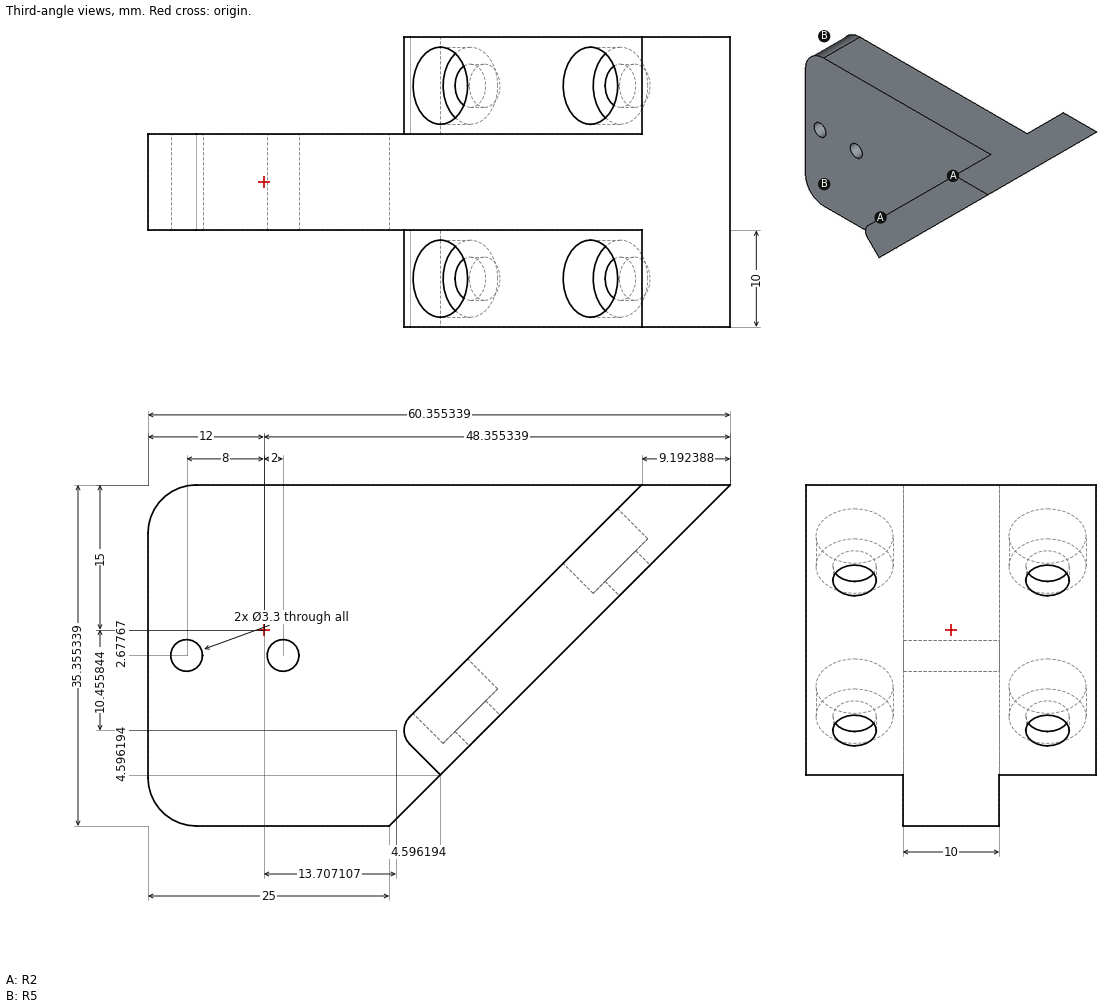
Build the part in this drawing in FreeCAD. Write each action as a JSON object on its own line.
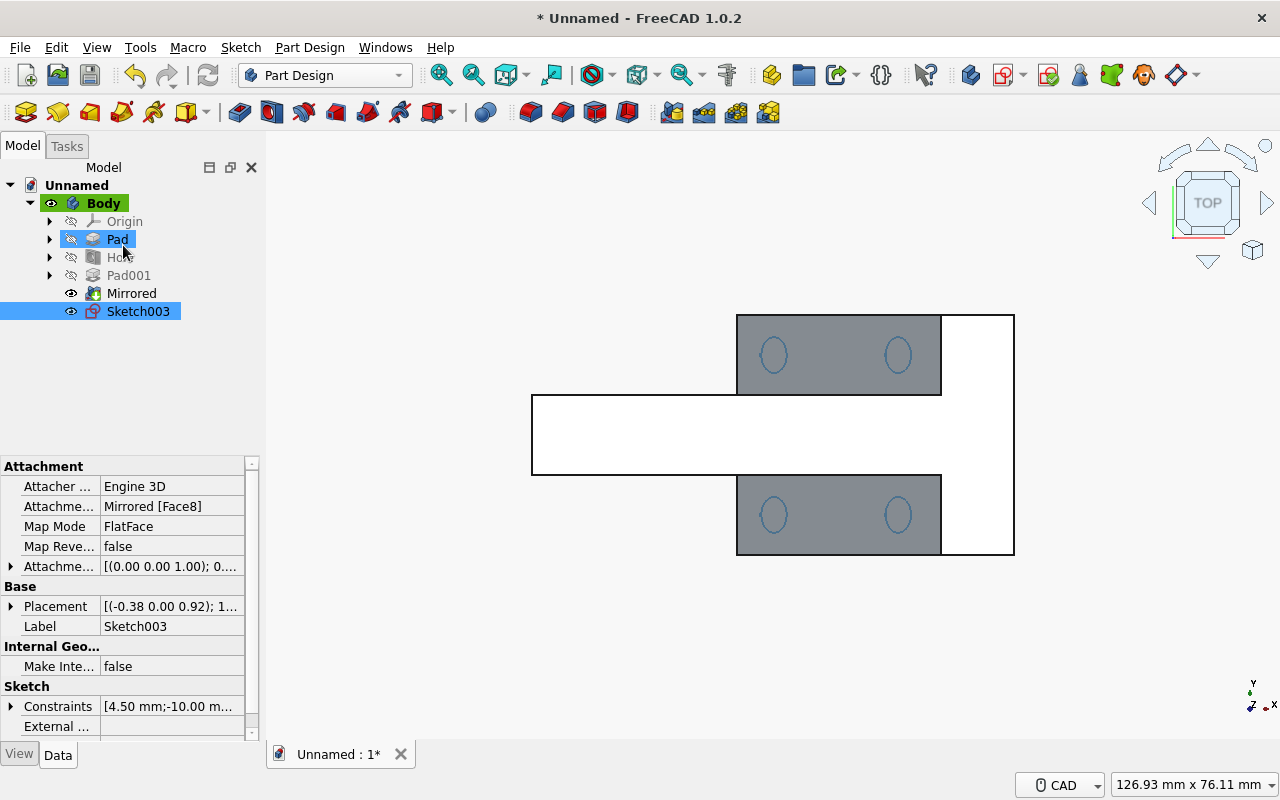
{"action": "left_click", "coordinate": [272, 112]}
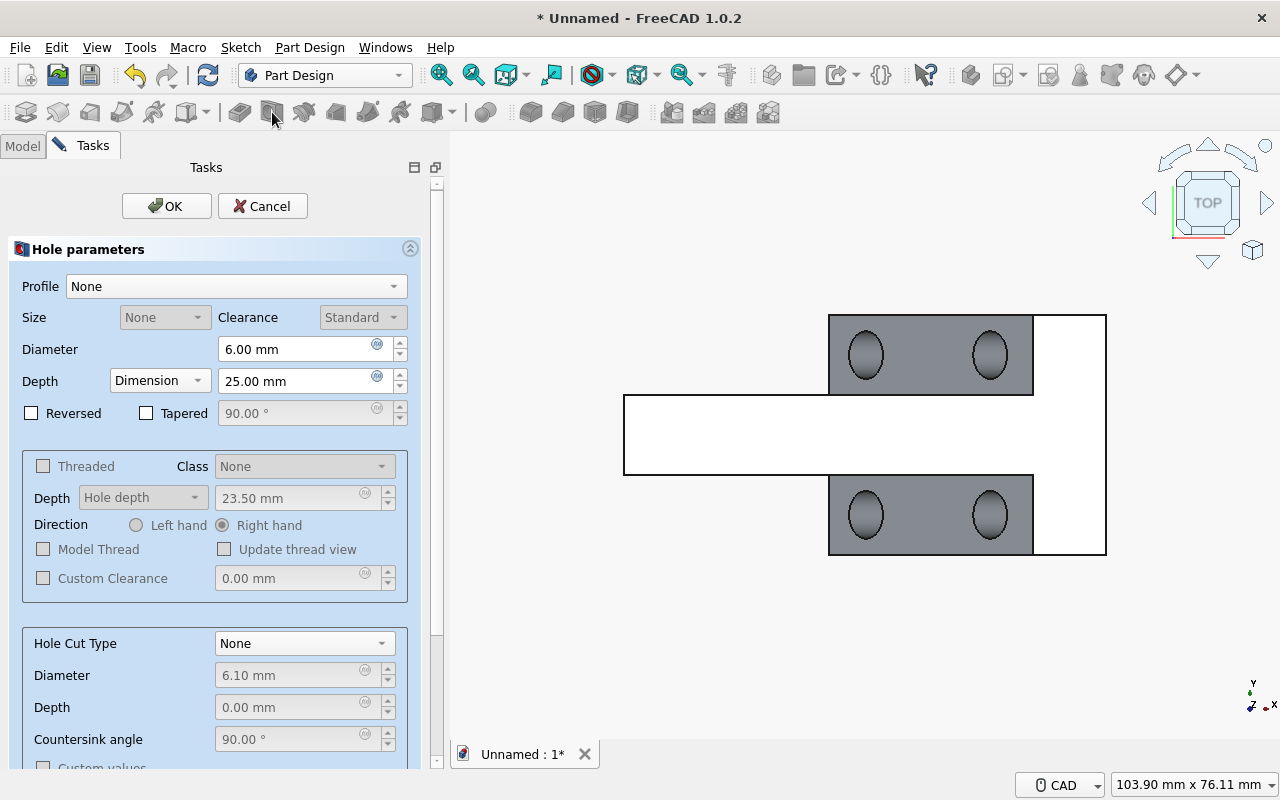
{"action": "triple_click", "coordinate": [305, 349]}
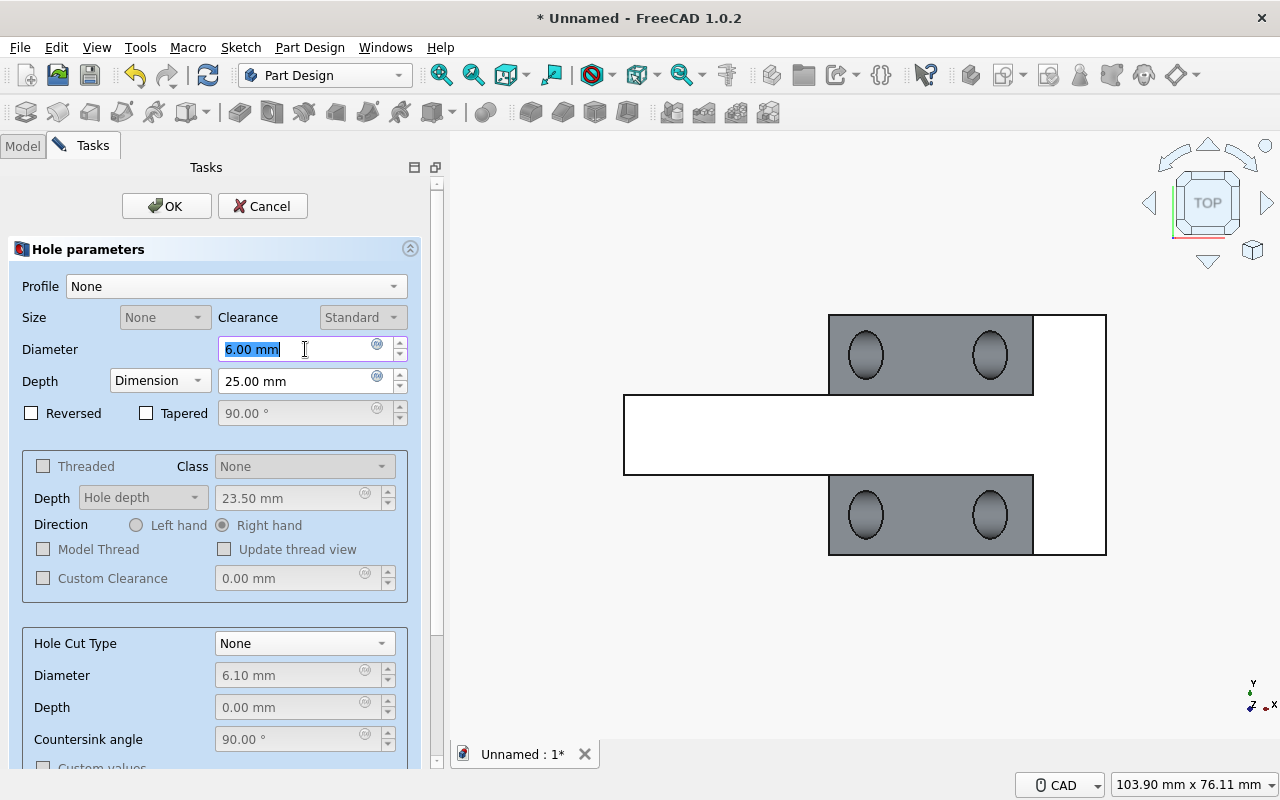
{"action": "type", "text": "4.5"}
{"action": "key", "text": "Tab"}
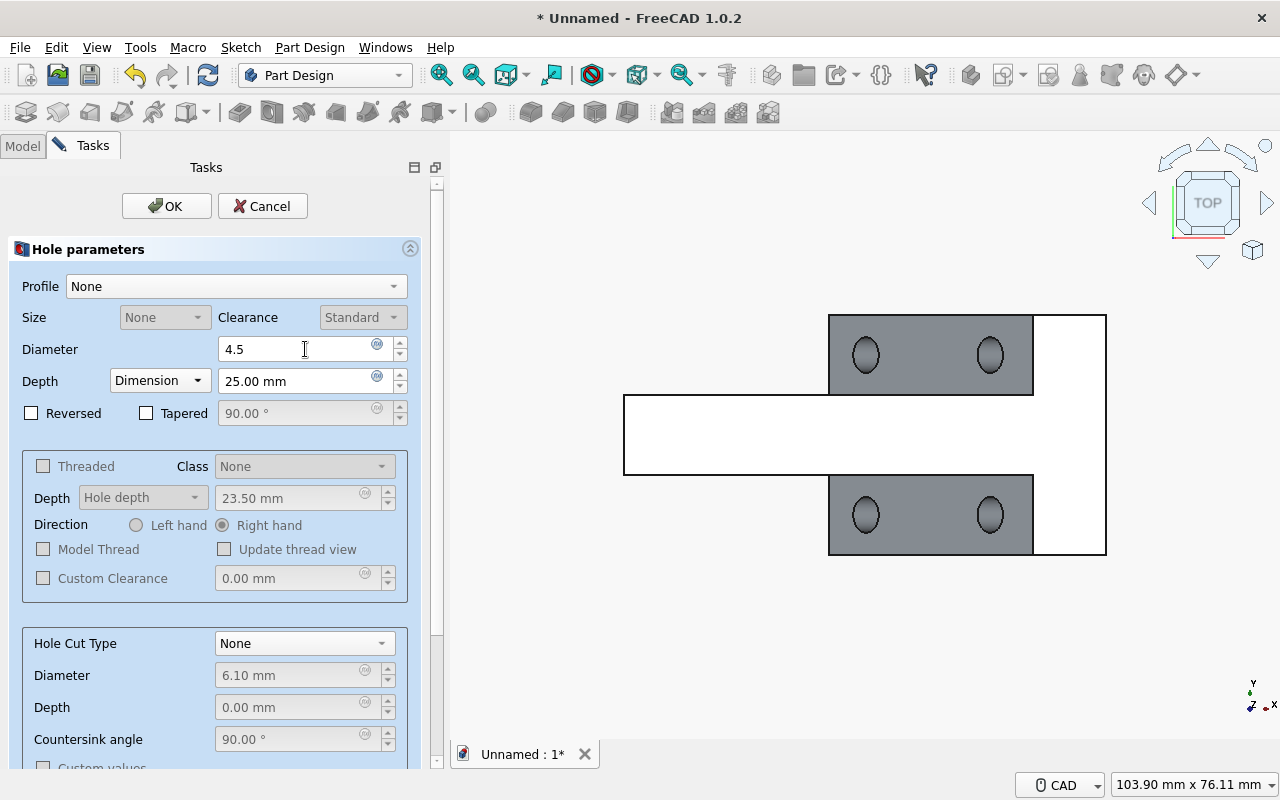
{"action": "left_click", "coordinate": [161, 380]}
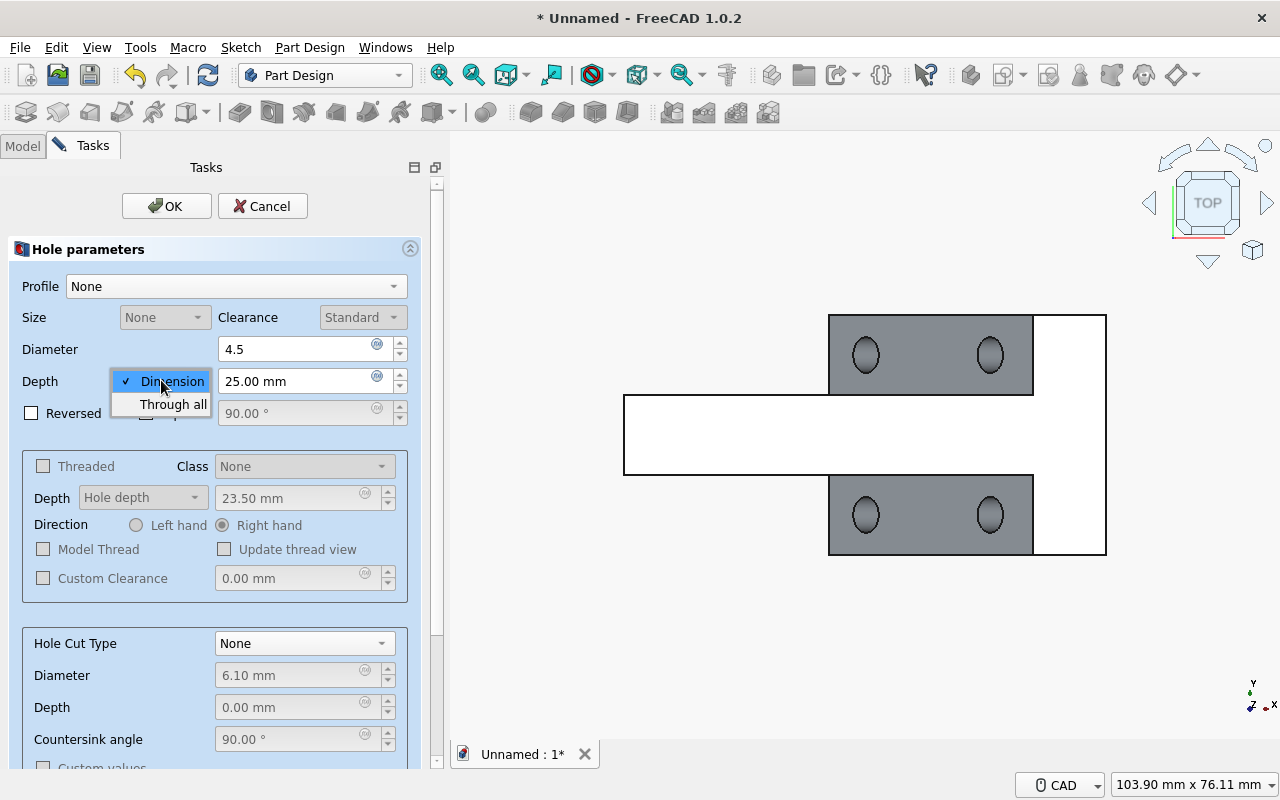
{"action": "left_click", "coordinate": [160, 404]}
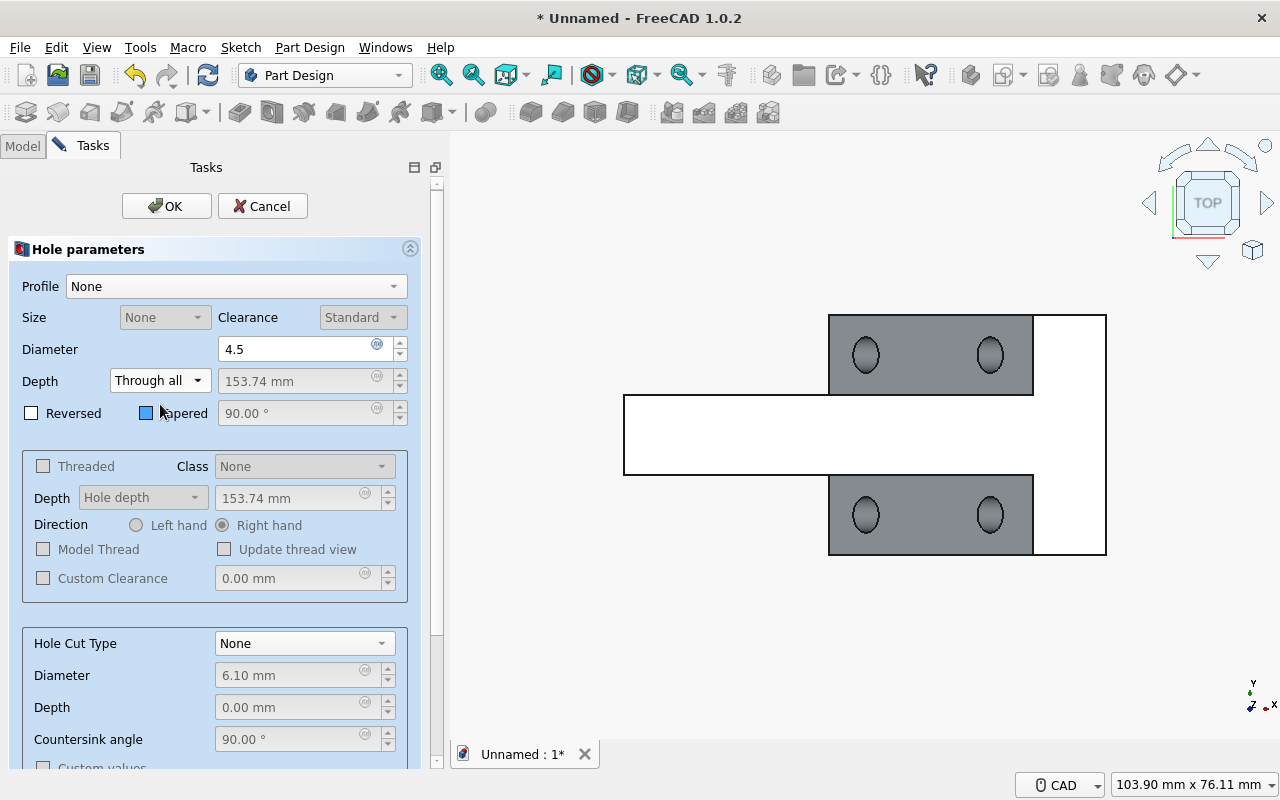
{"action": "left_click", "coordinate": [306, 644]}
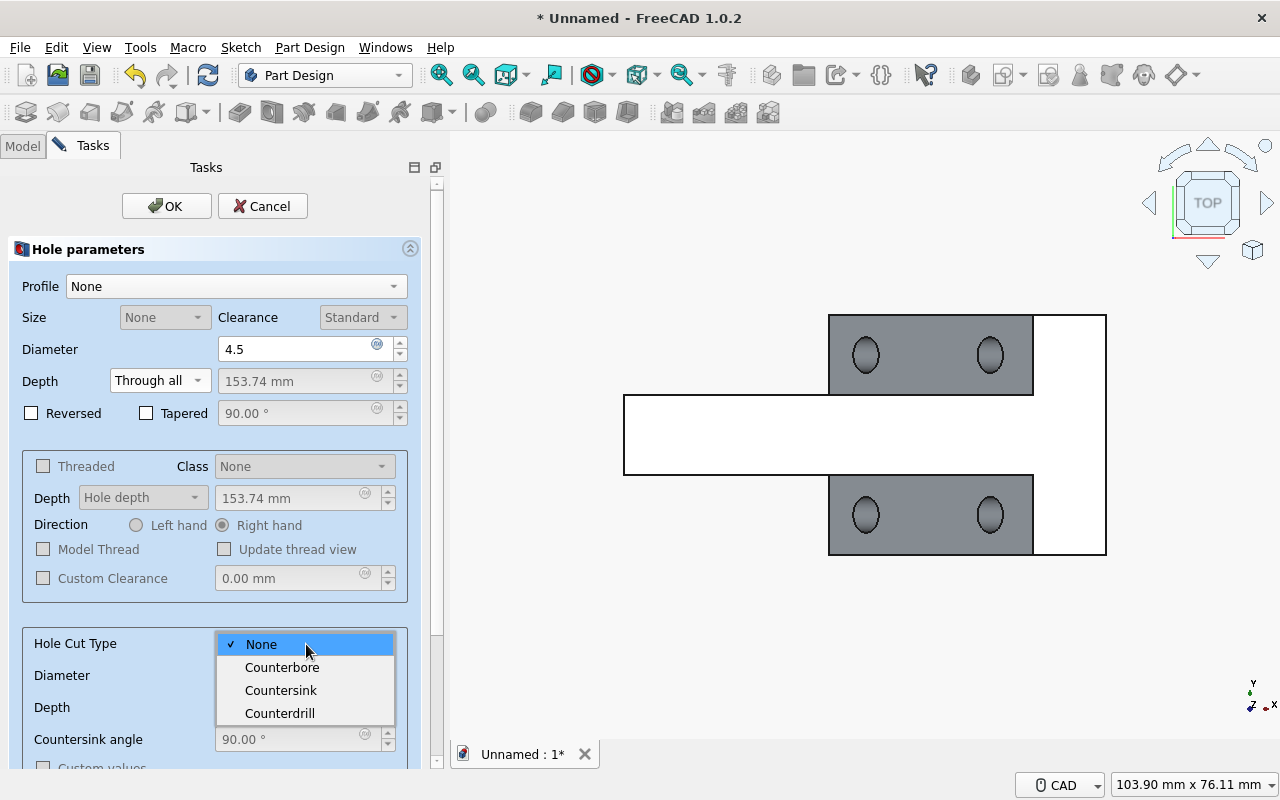
{"action": "left_click", "coordinate": [304, 668]}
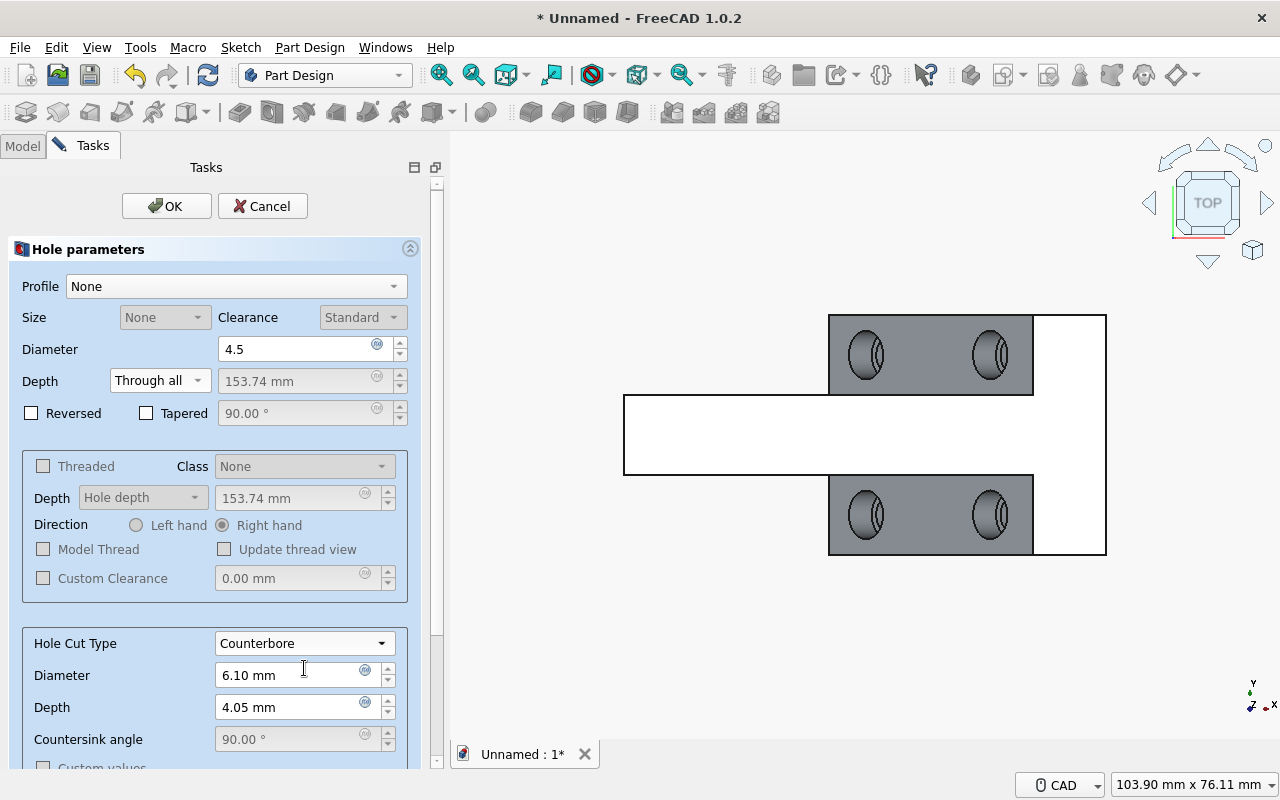
{"action": "triple_click", "coordinate": [298, 675]}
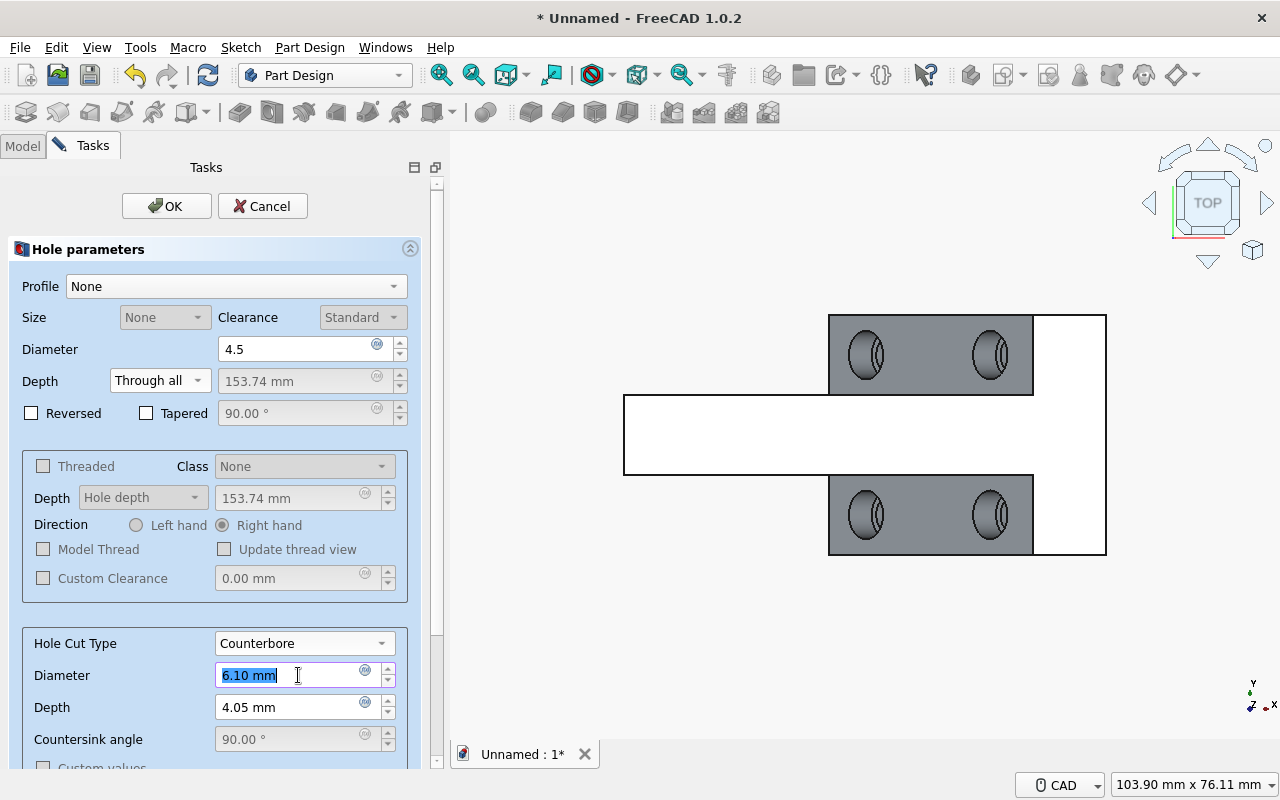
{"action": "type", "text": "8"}
{"action": "key", "text": "Tab"}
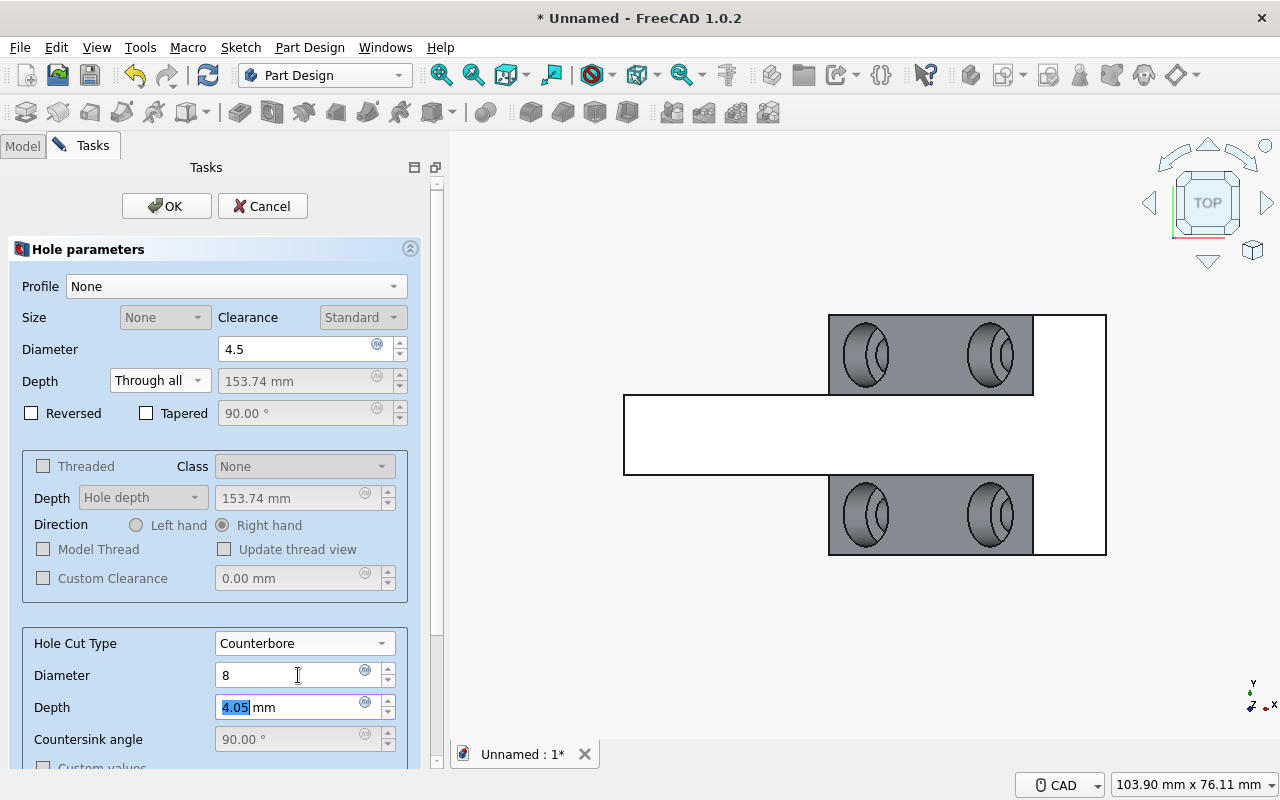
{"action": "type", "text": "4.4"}
{"action": "key", "text": "Tab"}